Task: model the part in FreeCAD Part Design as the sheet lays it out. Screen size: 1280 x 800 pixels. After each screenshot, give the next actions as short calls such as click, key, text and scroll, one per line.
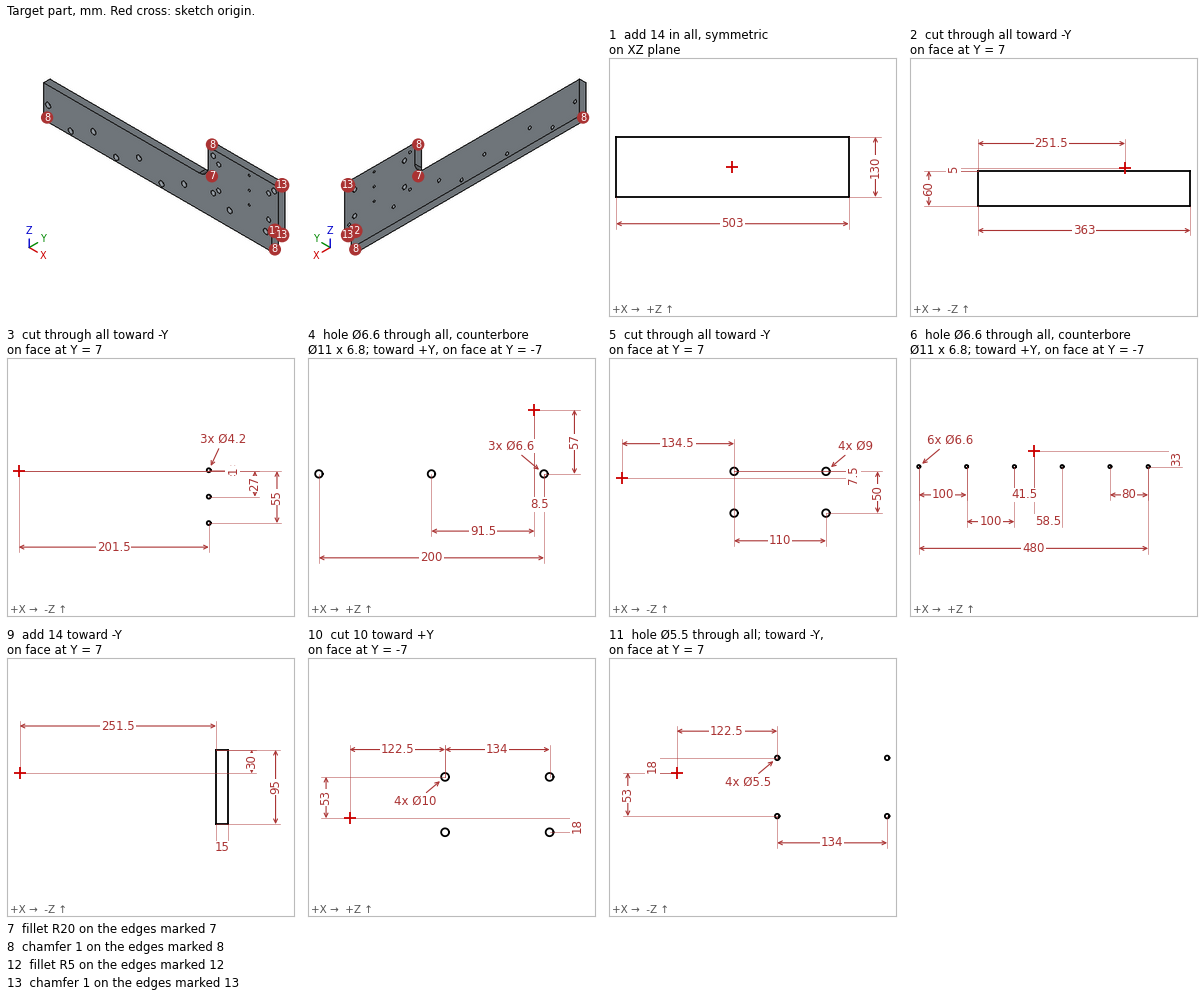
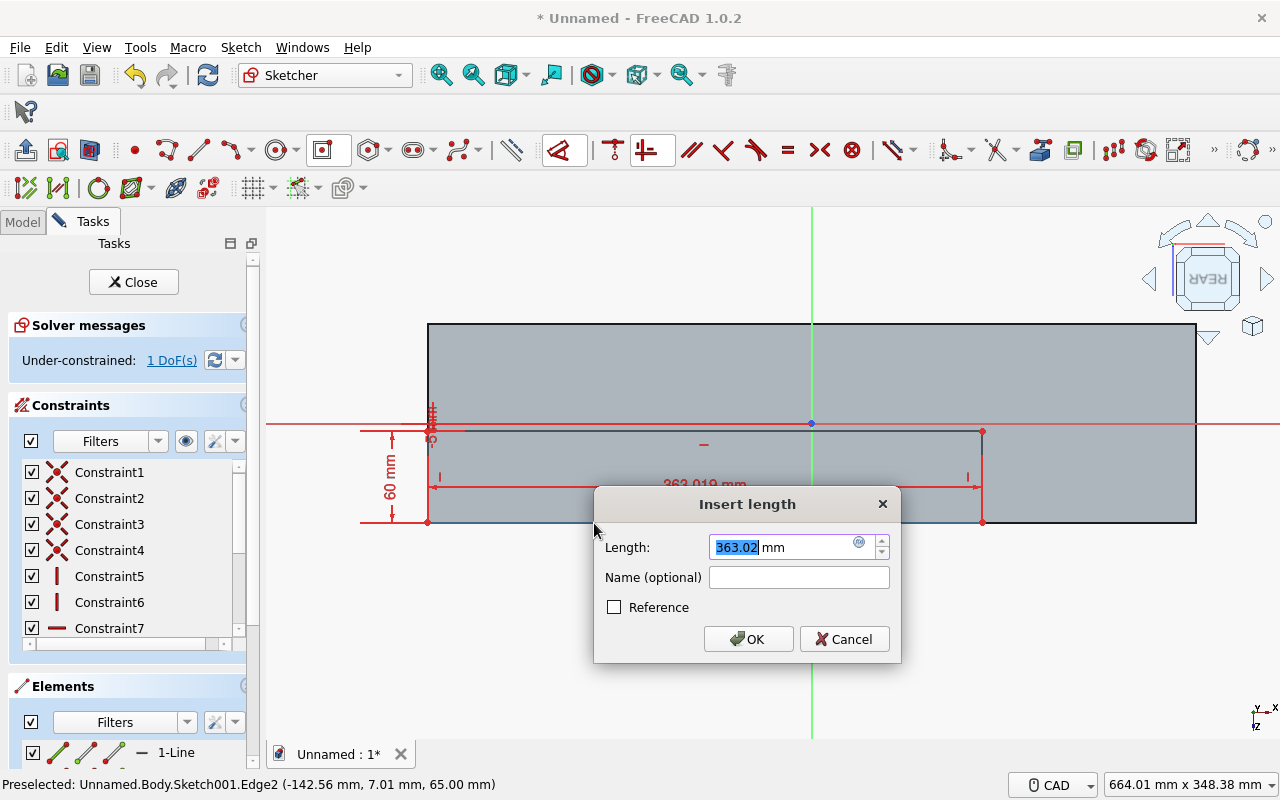
text(363)
key(Return)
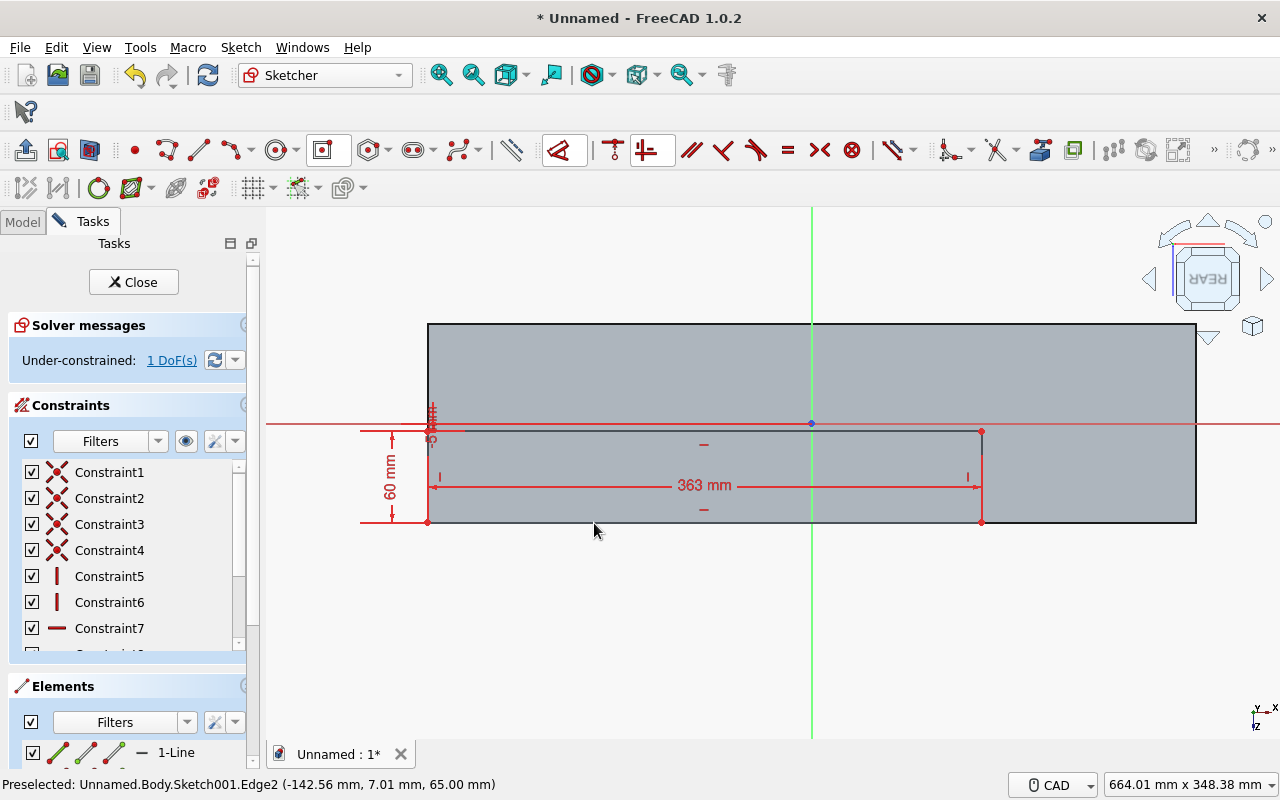
click(428, 431)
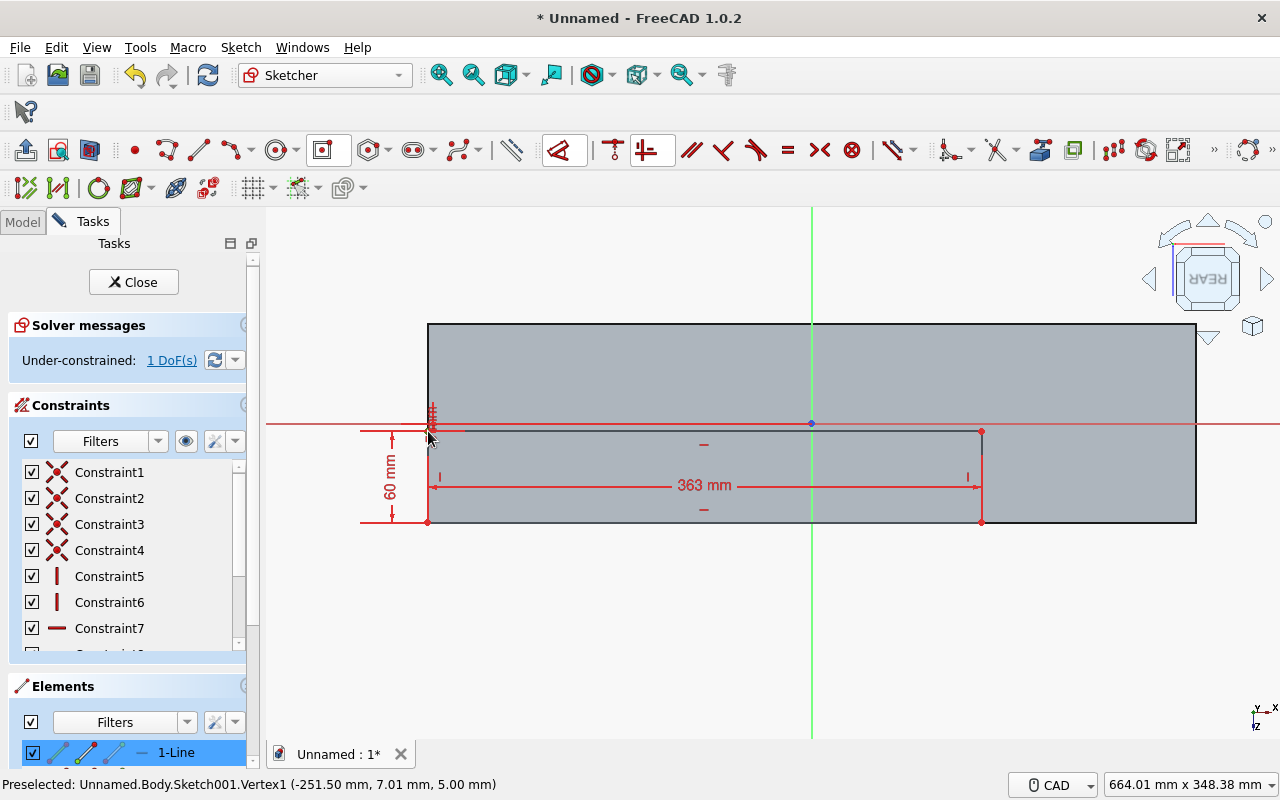
key(l)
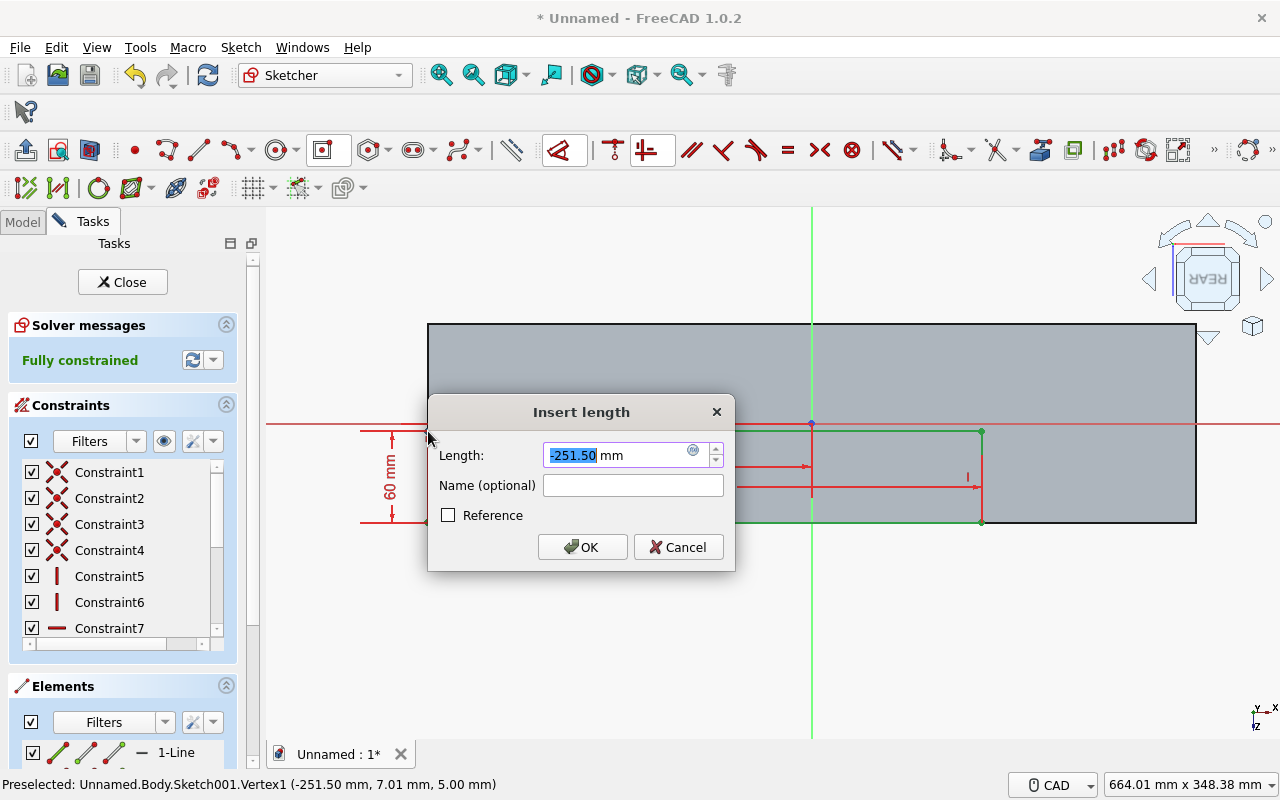
text(-251.5)
key(Return)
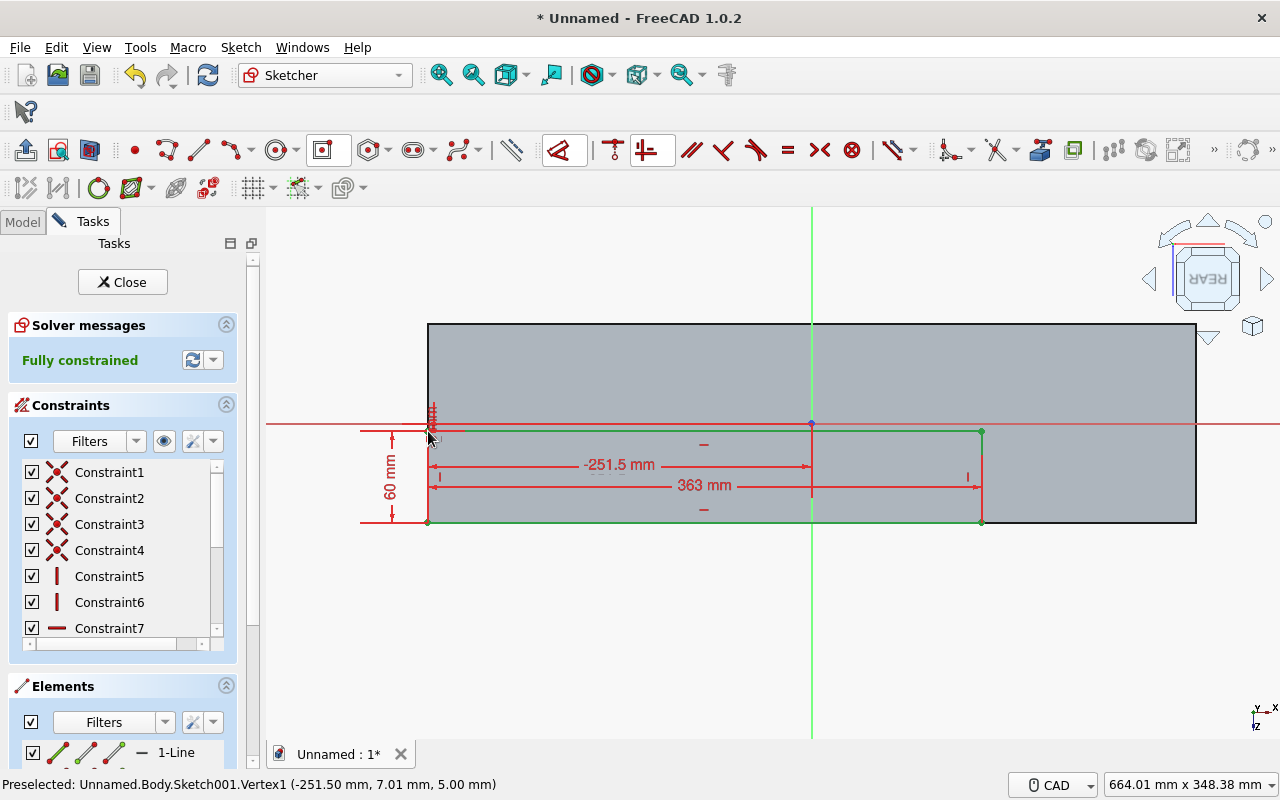
click(123, 282)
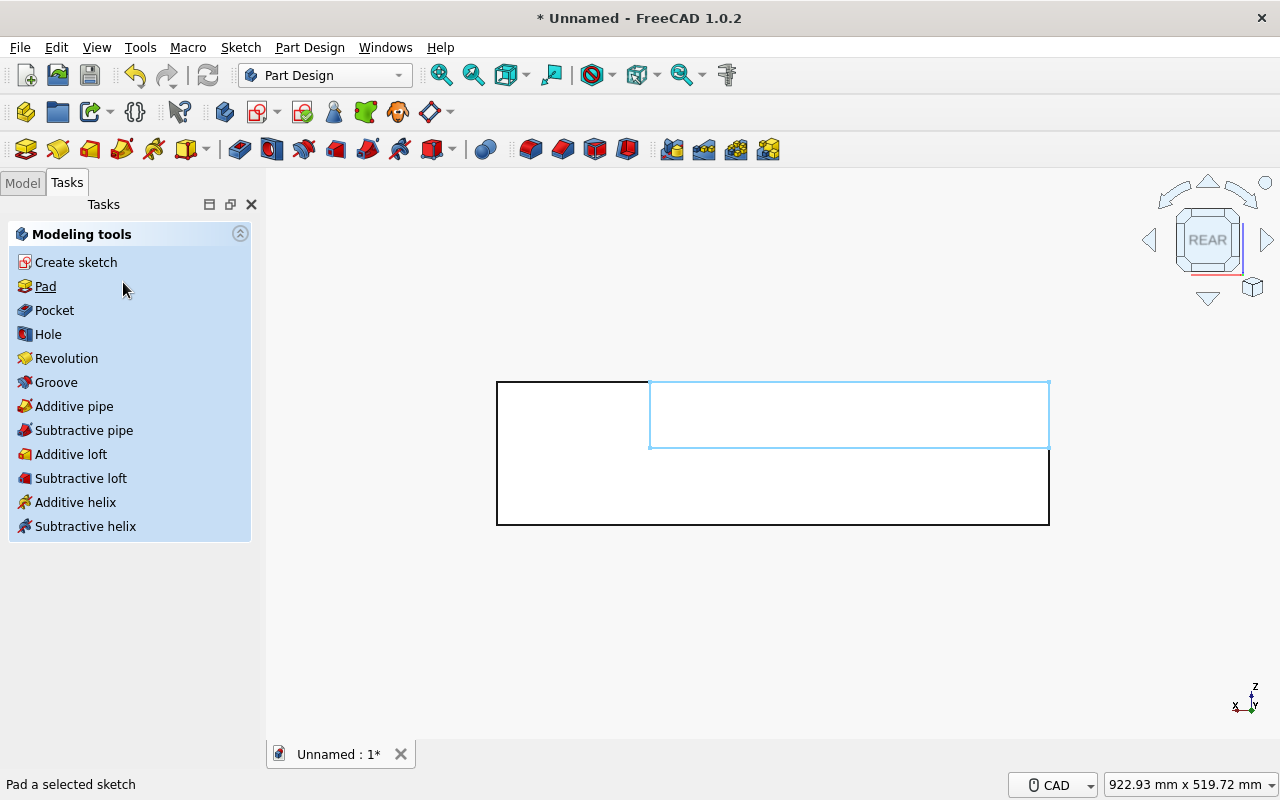
click(240, 150)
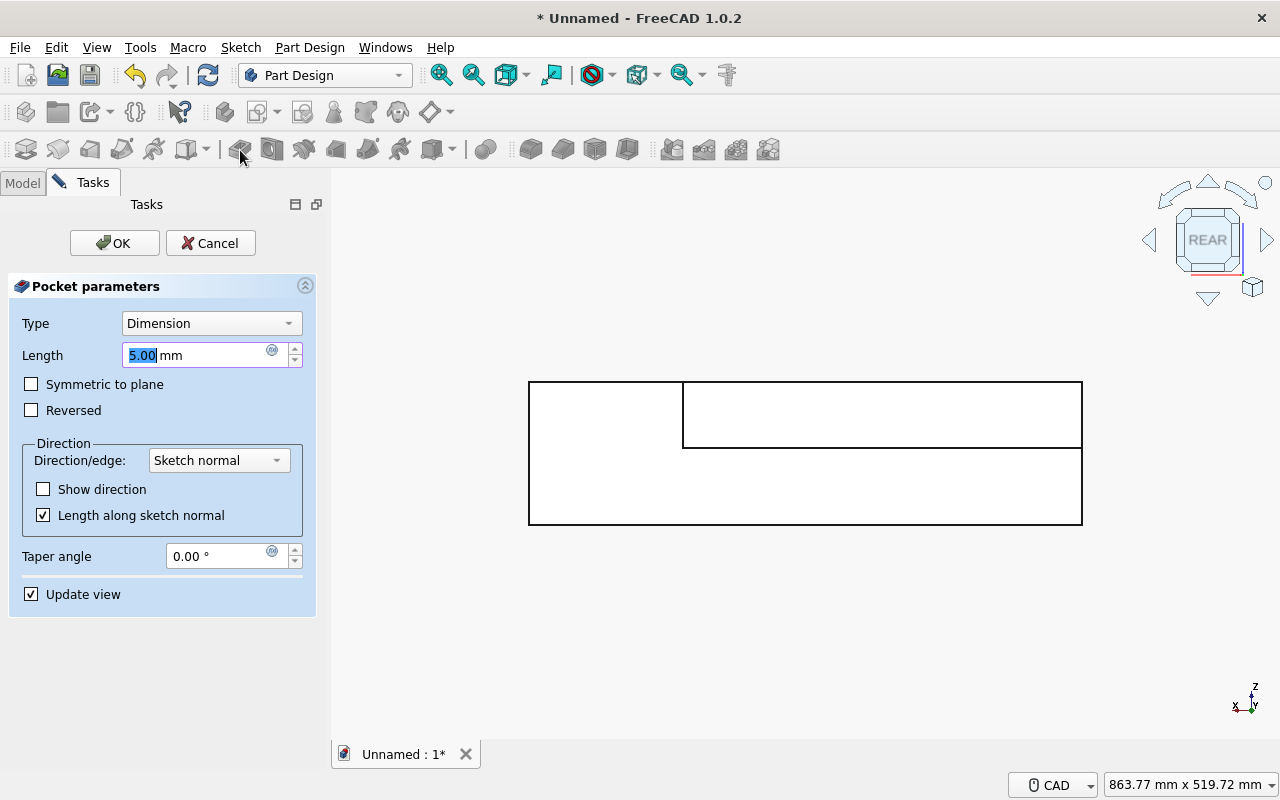
click(212, 324)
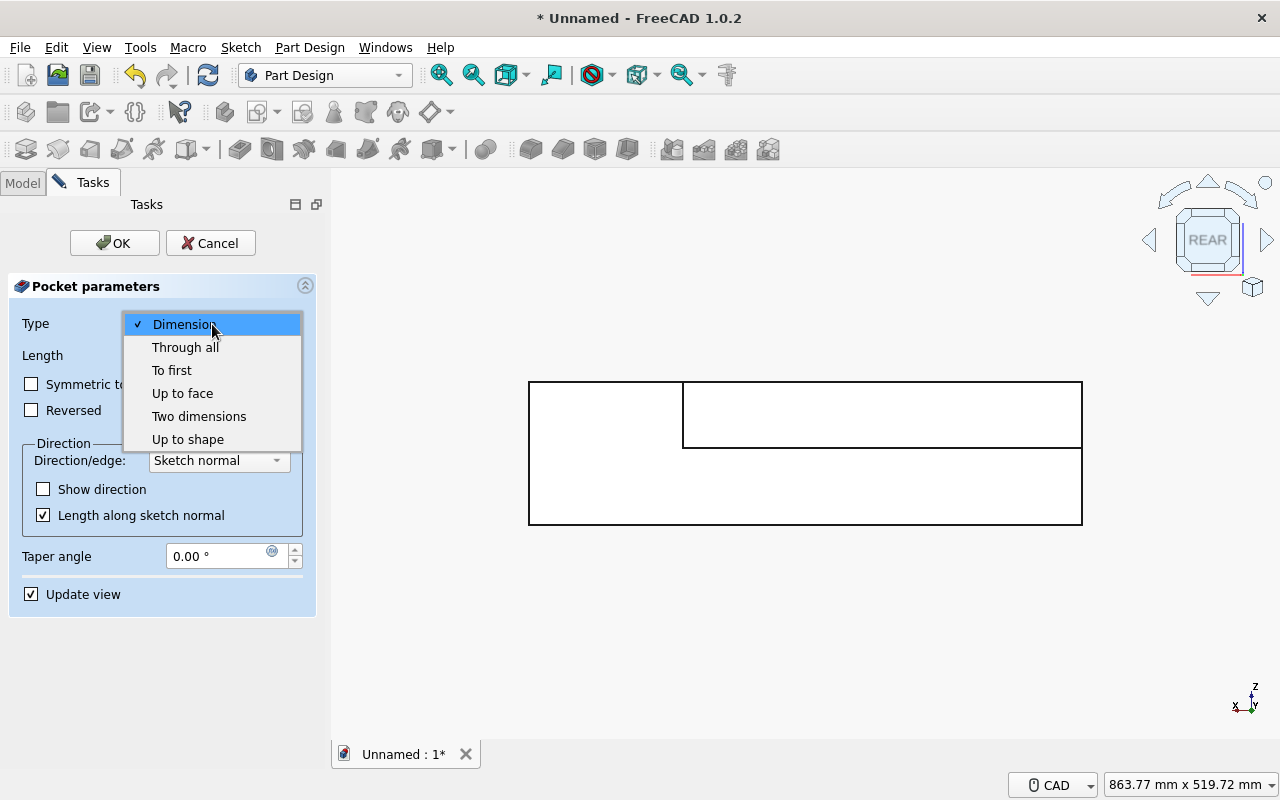
click(212, 348)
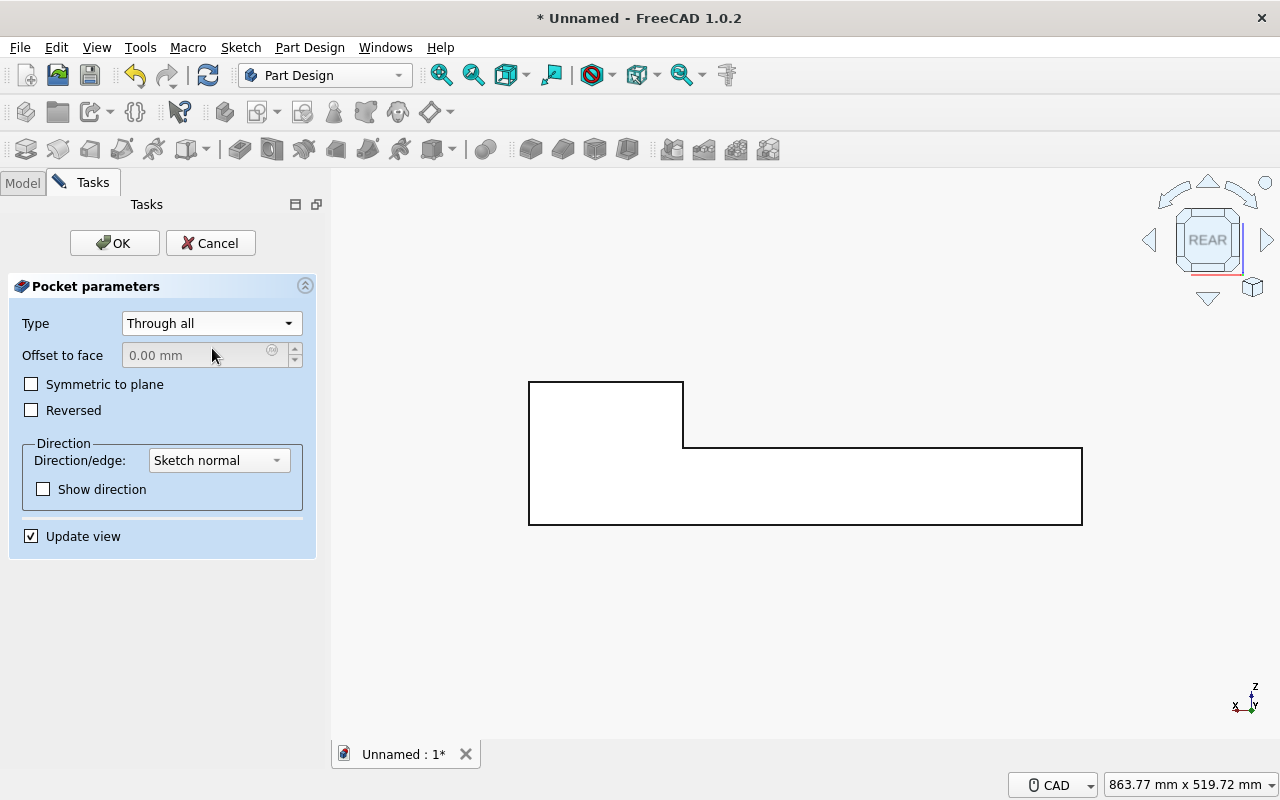
click(115, 243)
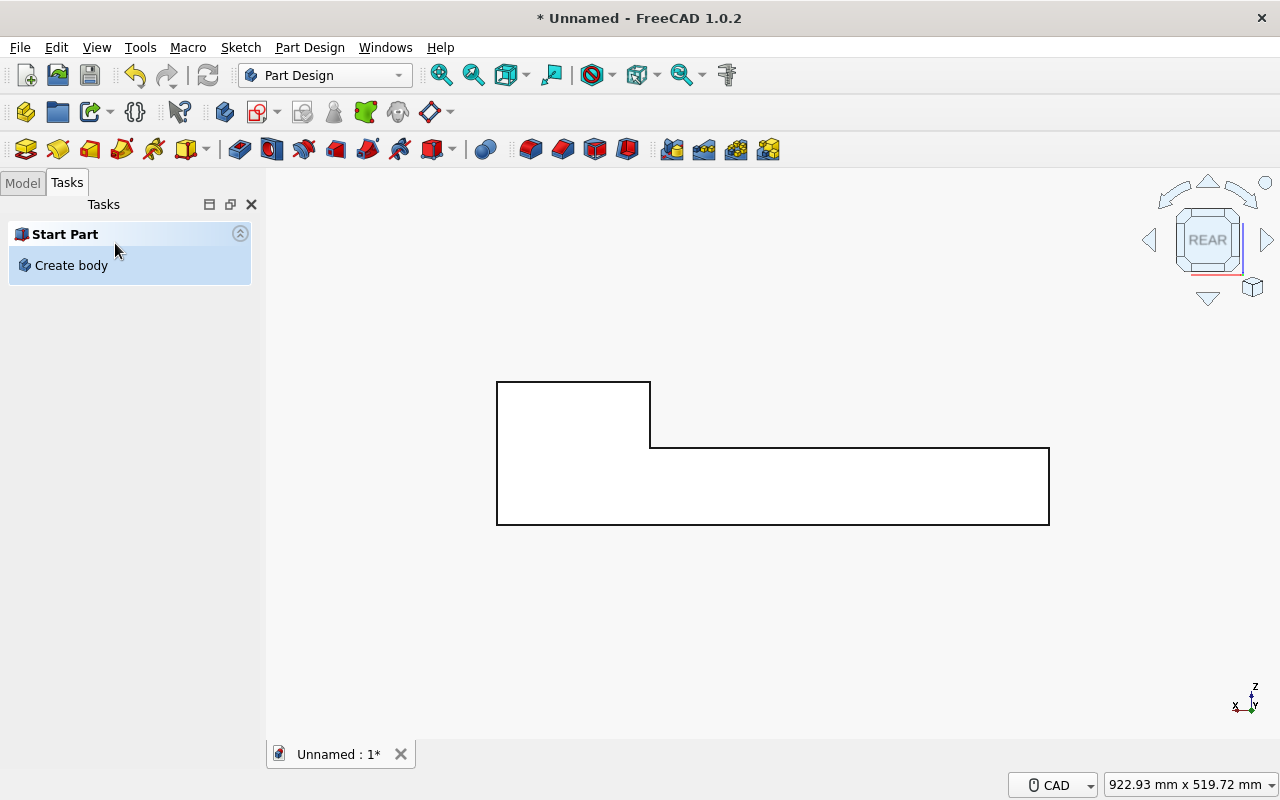
click(615, 473)